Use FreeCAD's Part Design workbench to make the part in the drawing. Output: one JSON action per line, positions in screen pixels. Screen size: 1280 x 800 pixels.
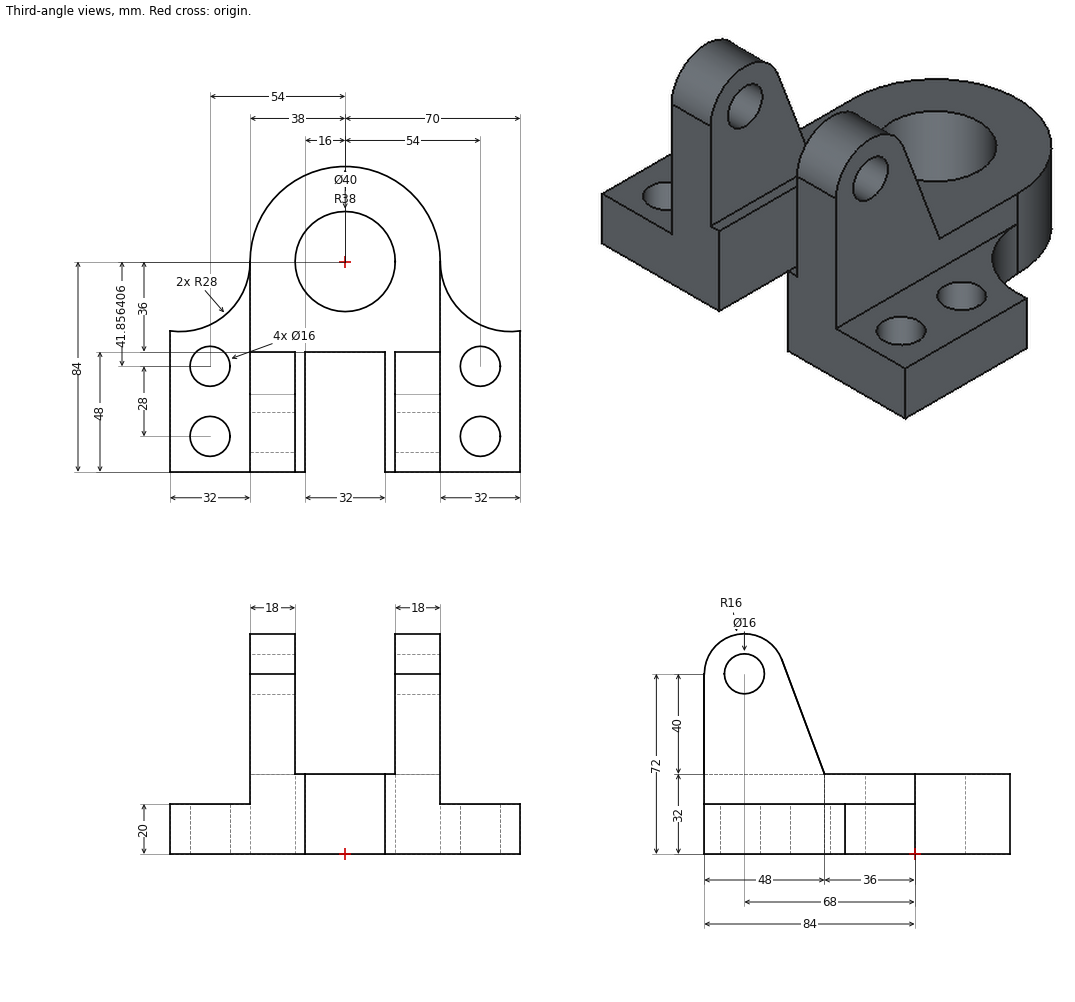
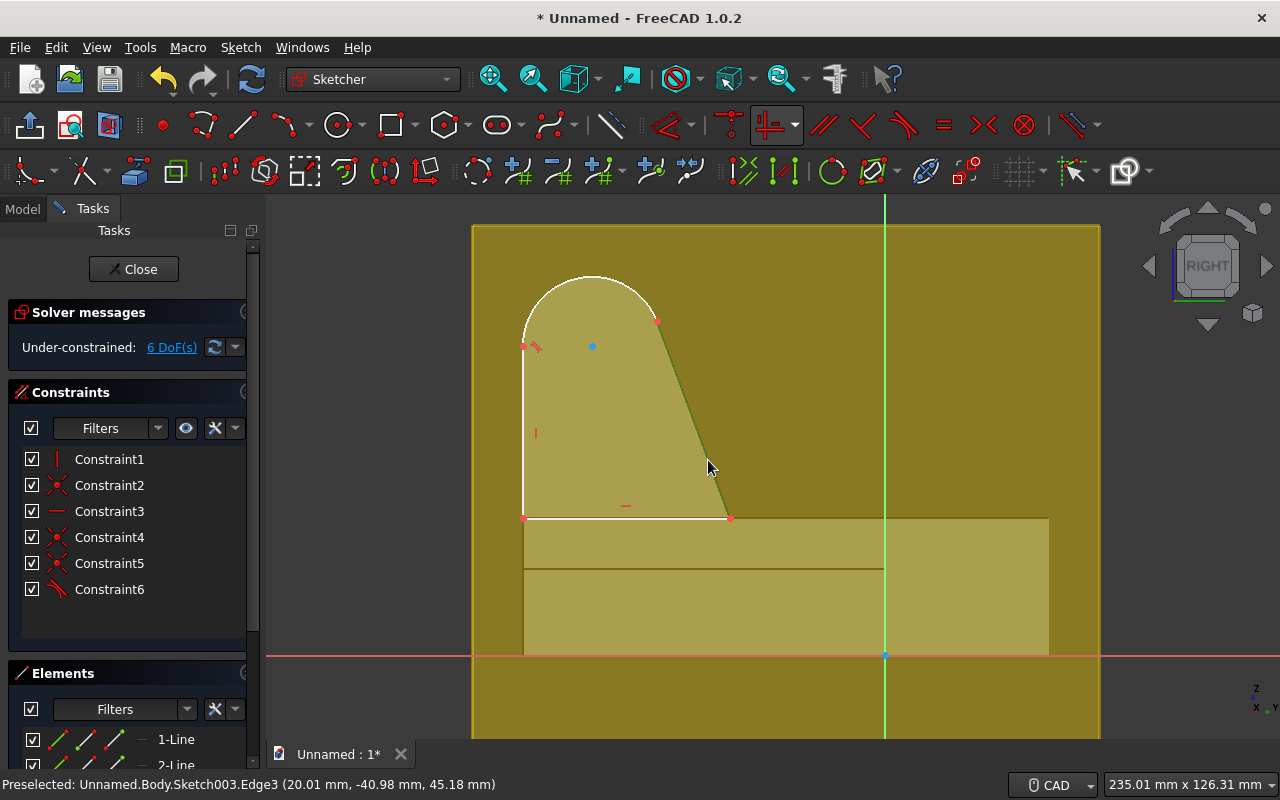
{"action": "left_click", "coordinate": [618, 282]}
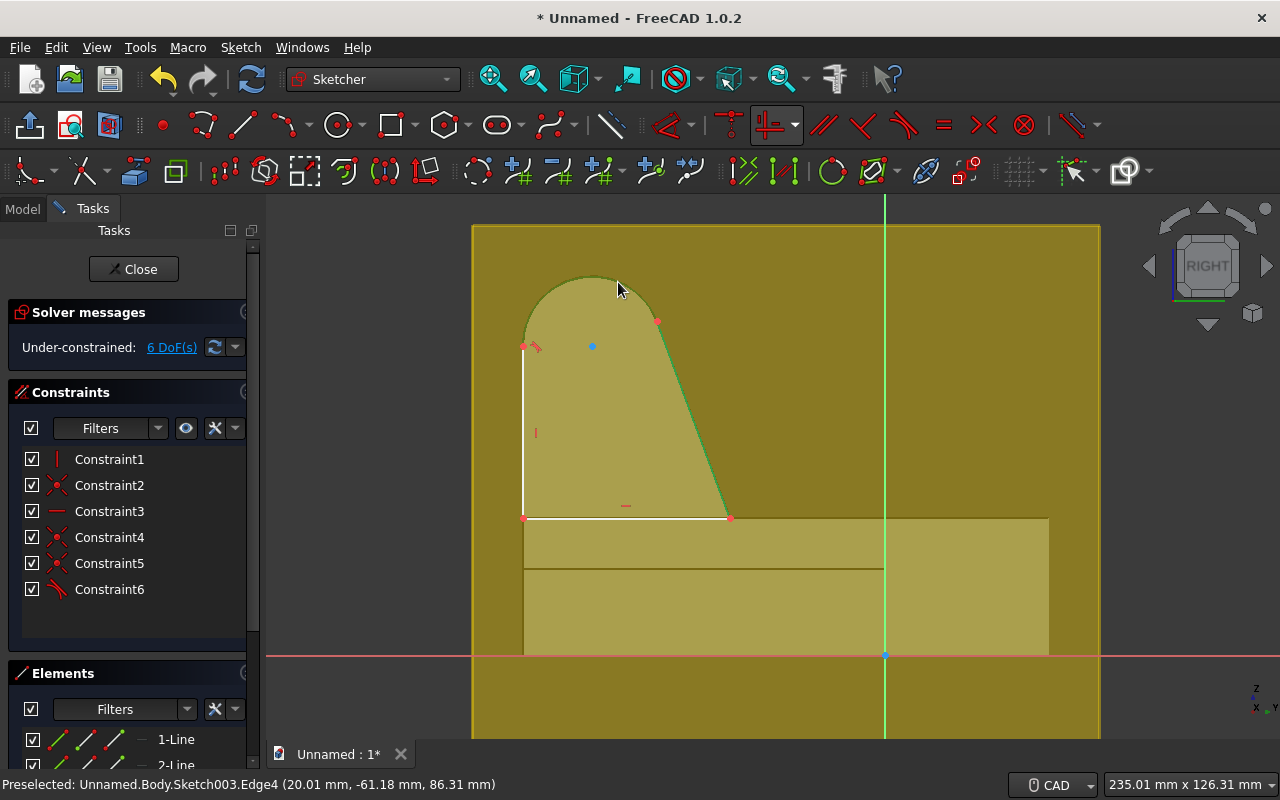
{"action": "left_click", "coordinate": [904, 126]}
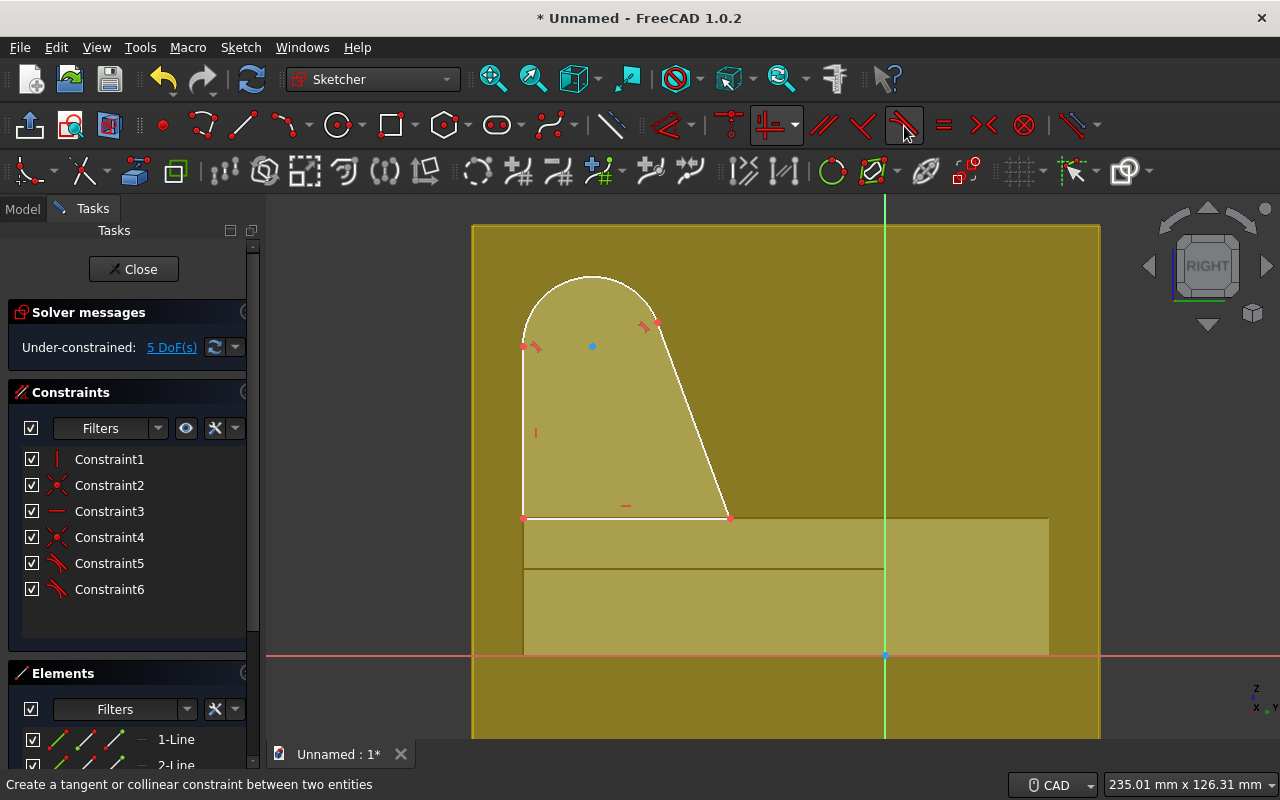
{"action": "left_click", "coordinate": [666, 126]}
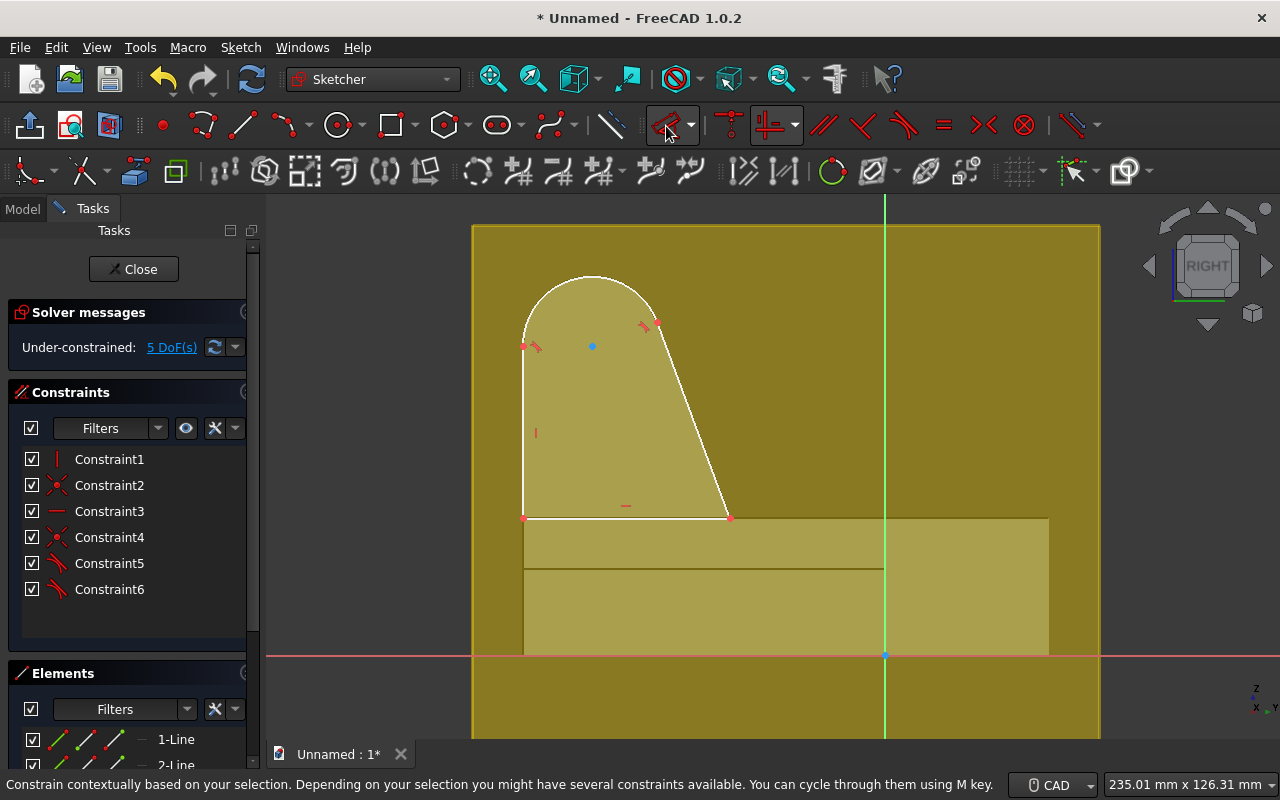
{"action": "left_click", "coordinate": [618, 282]}
{"action": "left_click", "coordinate": [630, 252]}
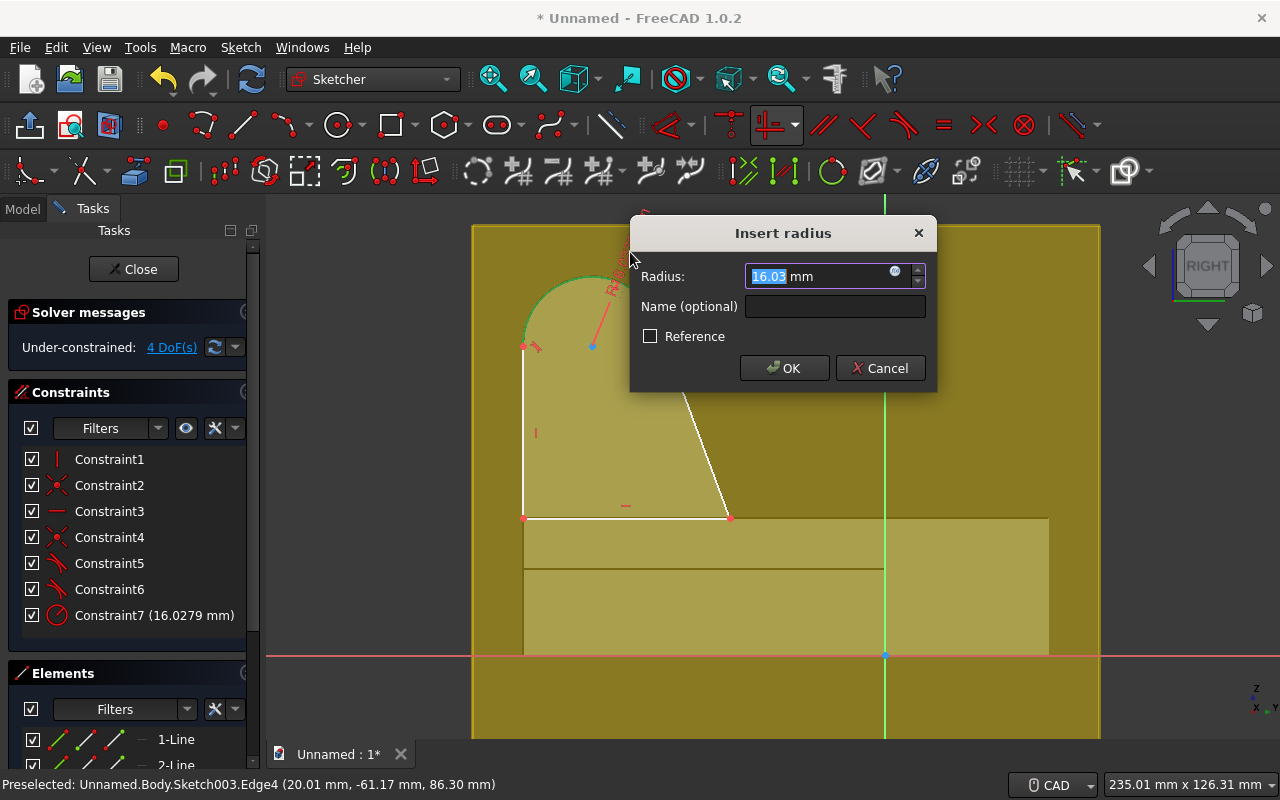
{"action": "type", "text": "16"}
{"action": "key", "text": "Return"}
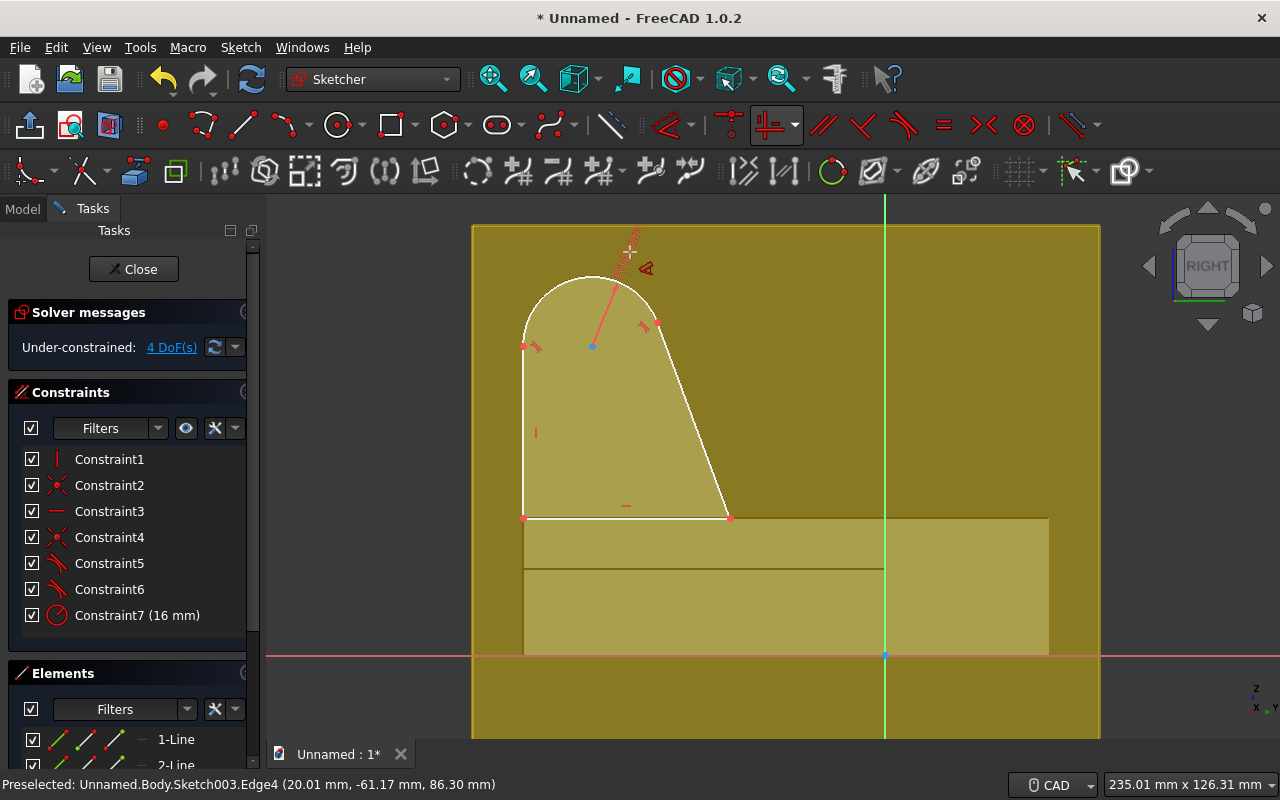
{"action": "left_click", "coordinate": [523, 398]}
{"action": "left_click", "coordinate": [489, 433]}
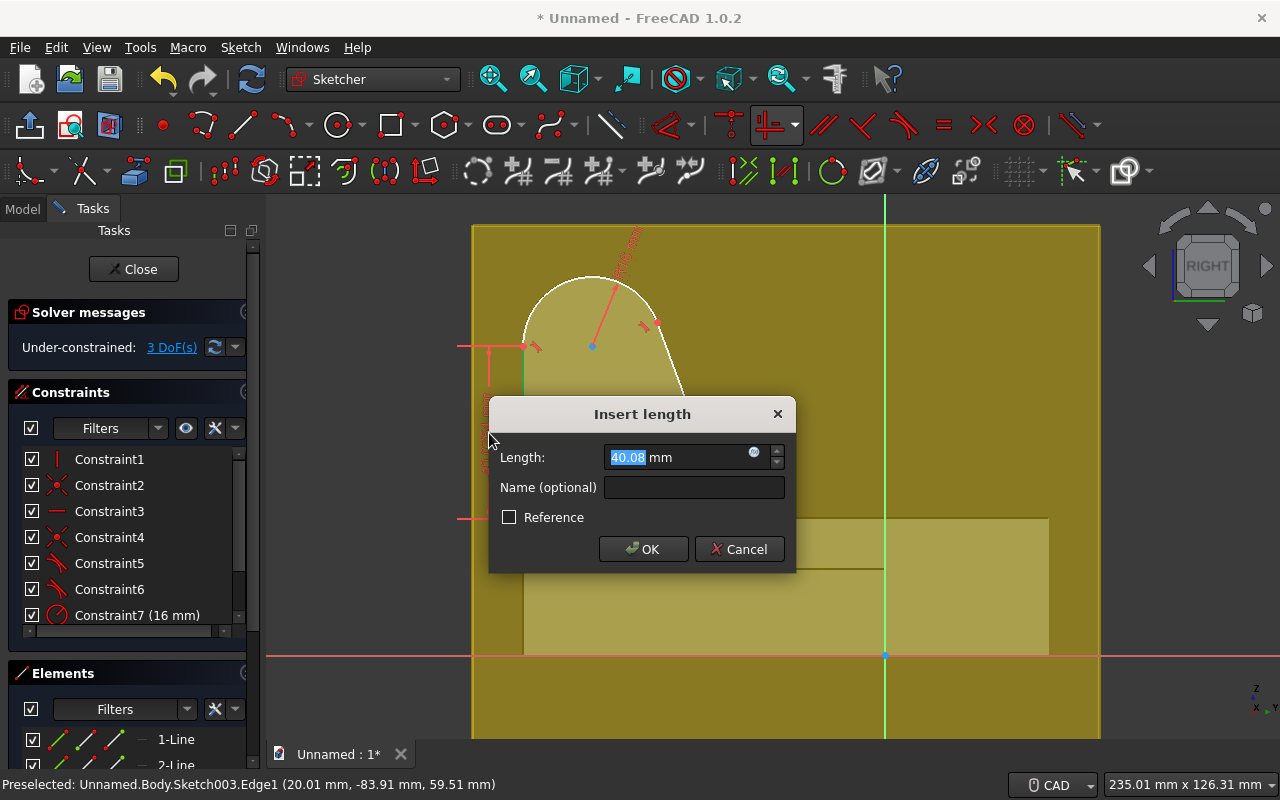
{"action": "type", "text": "40"}
{"action": "key", "text": "Return"}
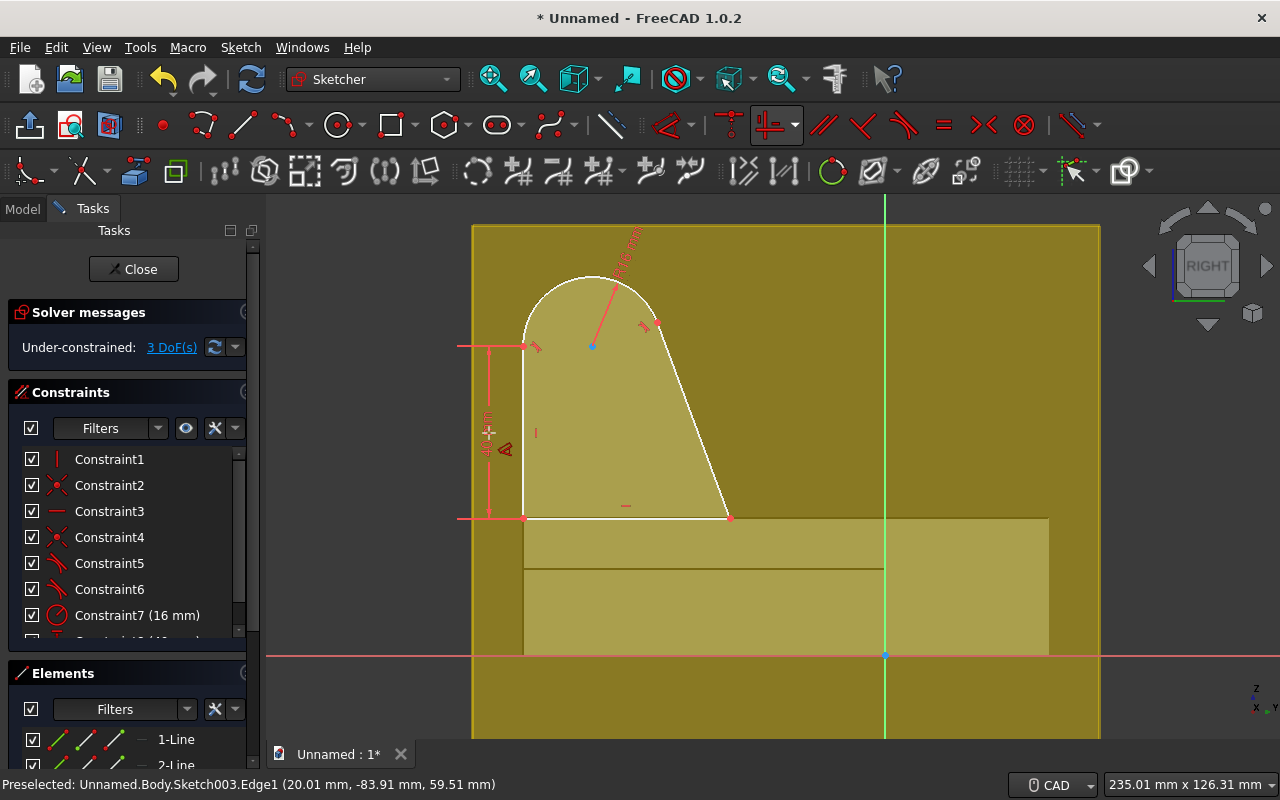
{"action": "left_click", "coordinate": [585, 519]}
{"action": "left_click", "coordinate": [627, 553]}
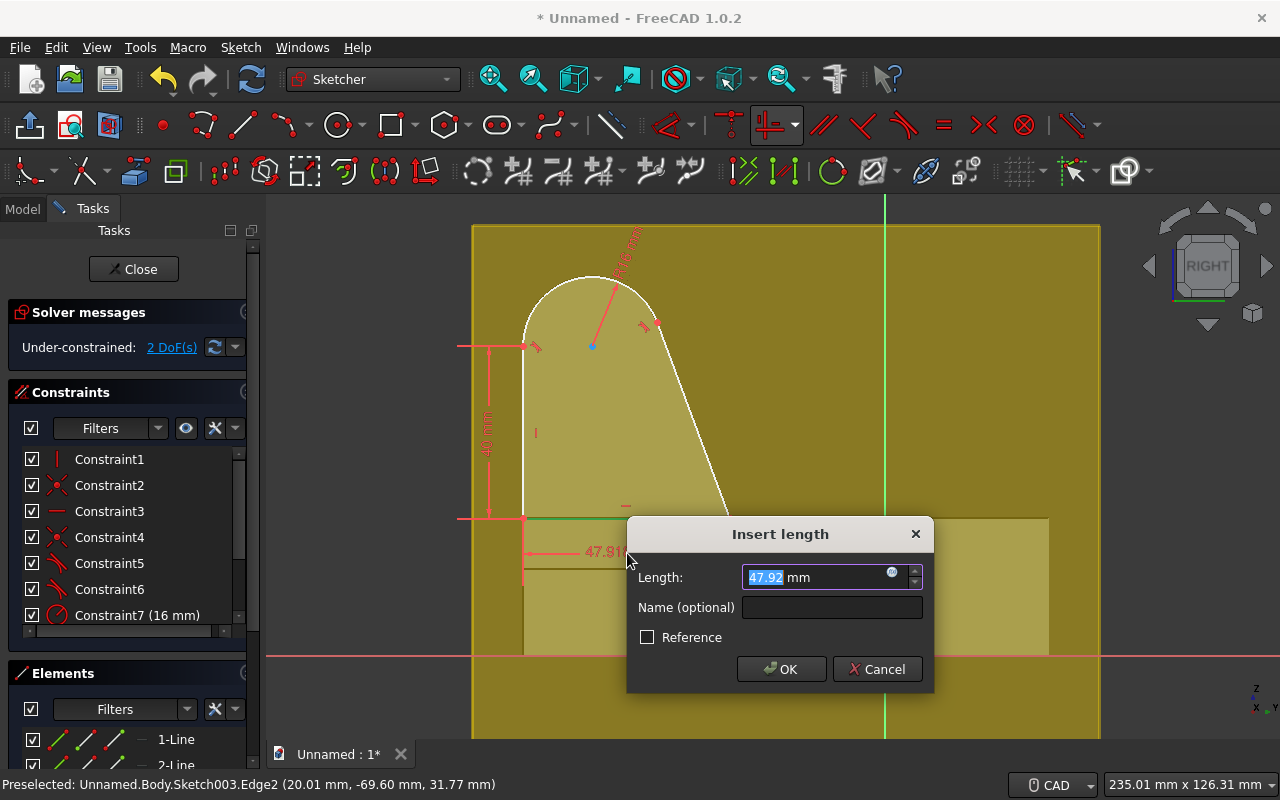
{"action": "type", "text": "48"}
{"action": "key", "text": "Return"}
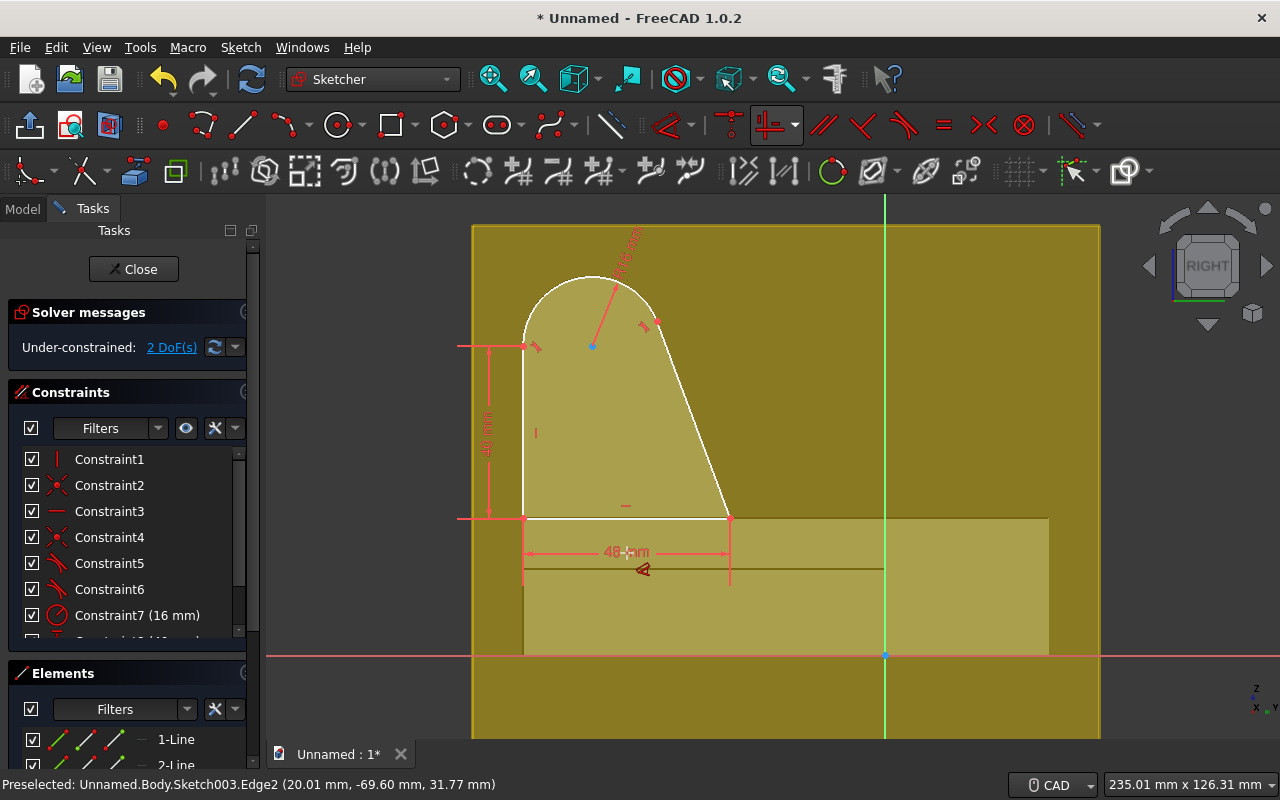
{"action": "left_click", "coordinate": [523, 346]}
{"action": "left_click", "coordinate": [704, 690]}